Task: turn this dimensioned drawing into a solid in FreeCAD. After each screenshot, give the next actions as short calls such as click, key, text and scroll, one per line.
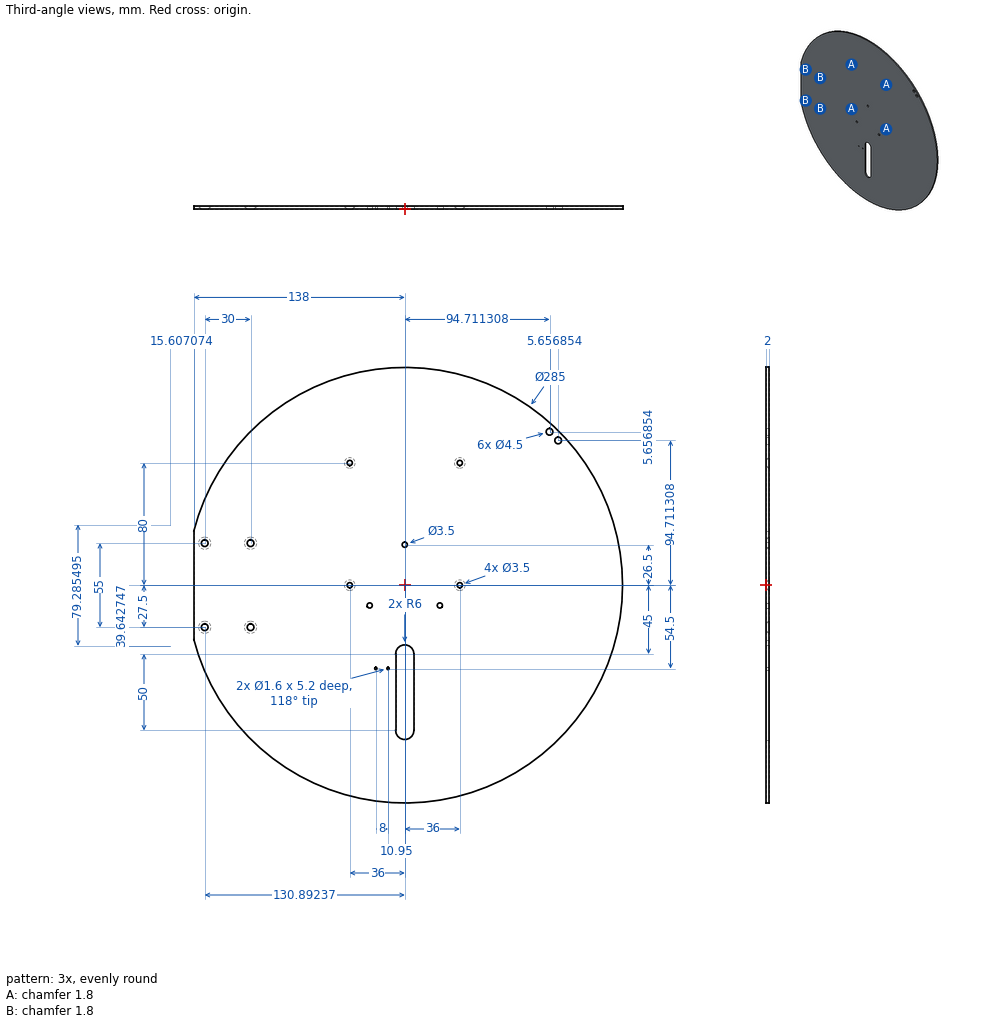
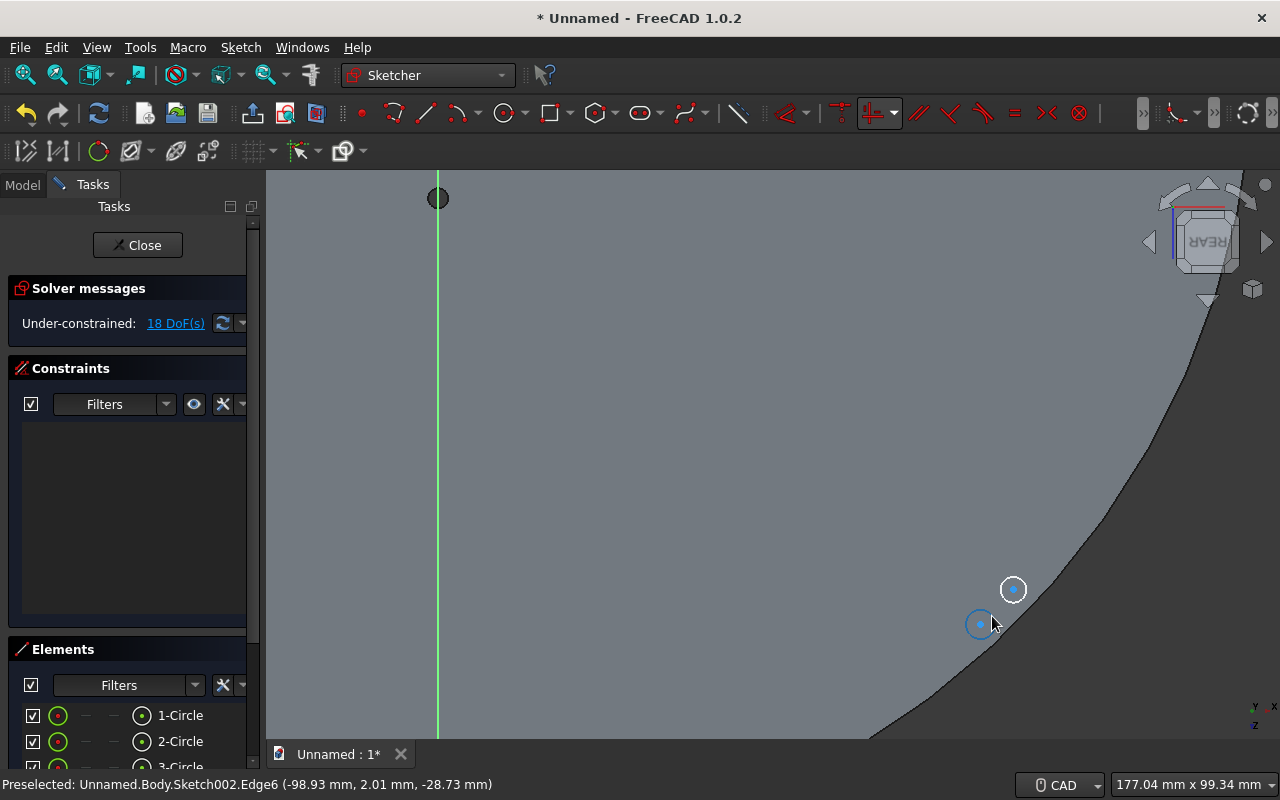
click(991, 614)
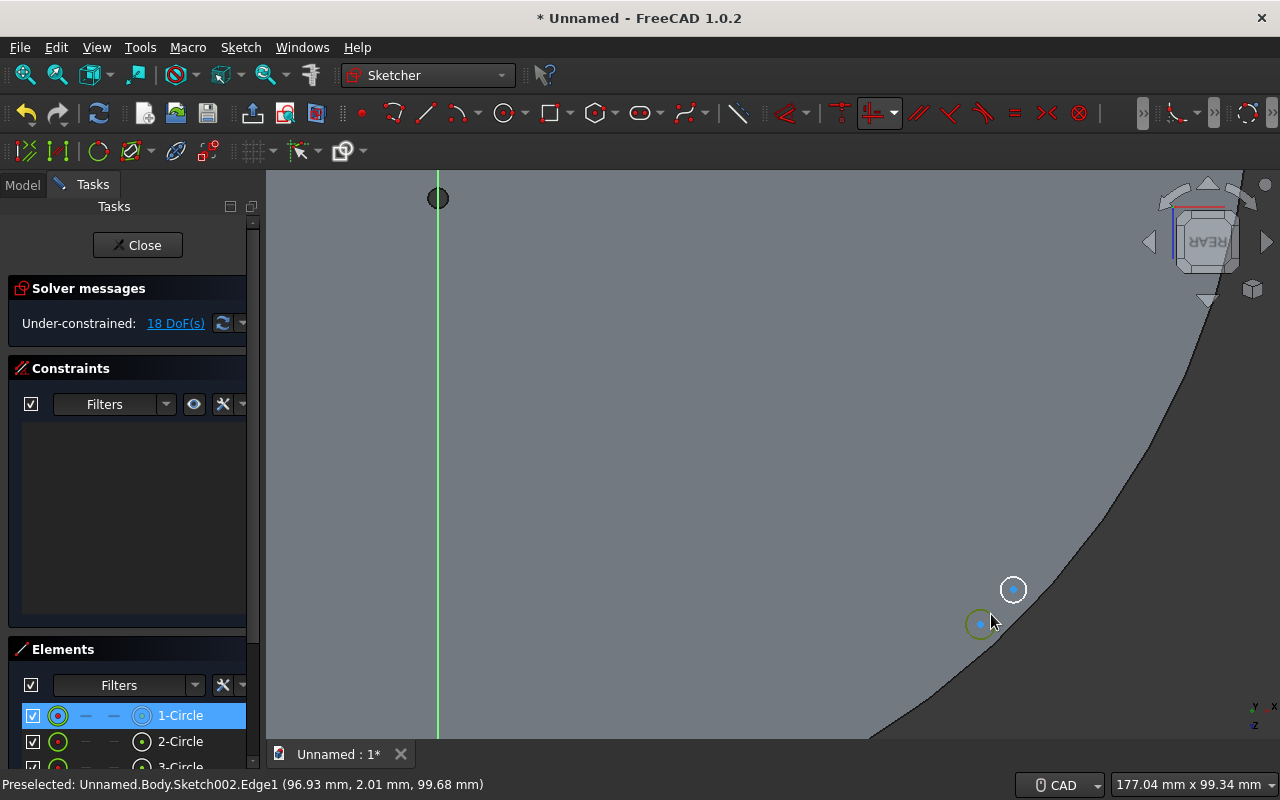
click(1022, 581)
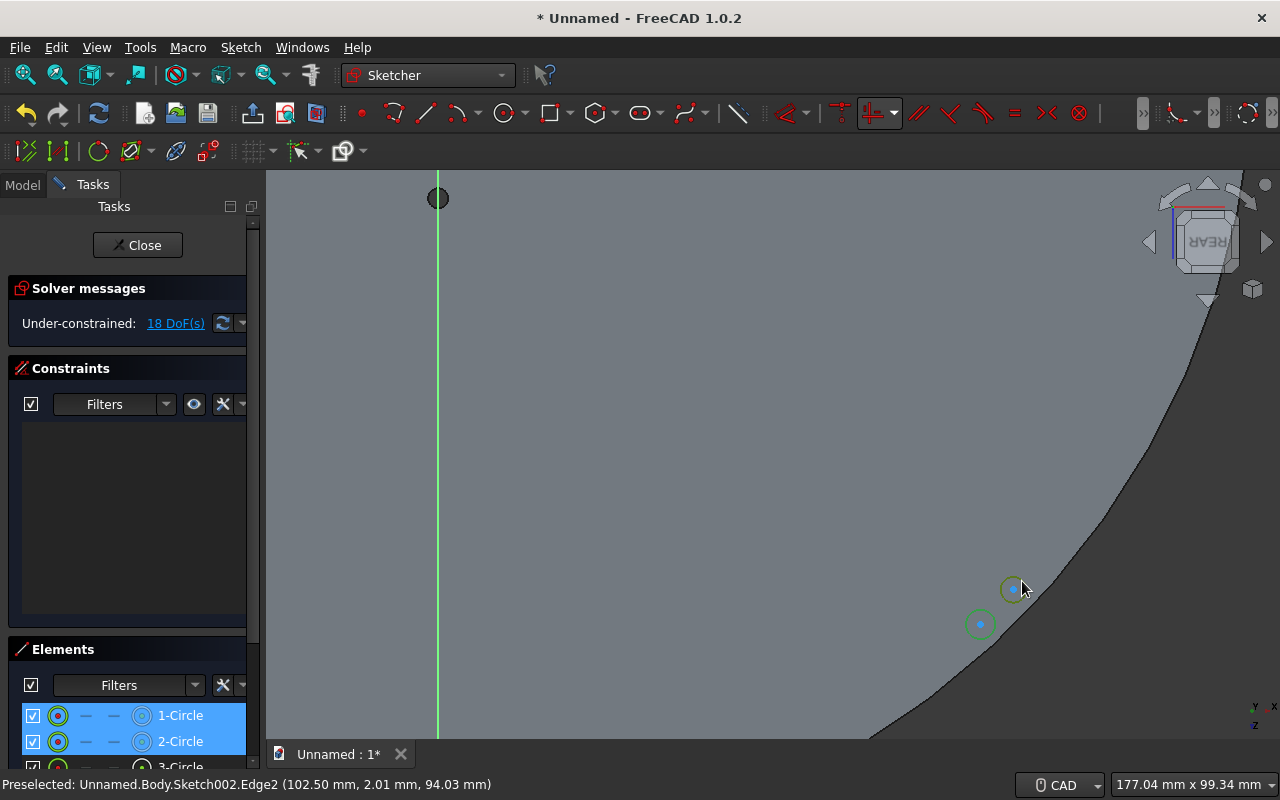
scroll(993, 617, down, 4)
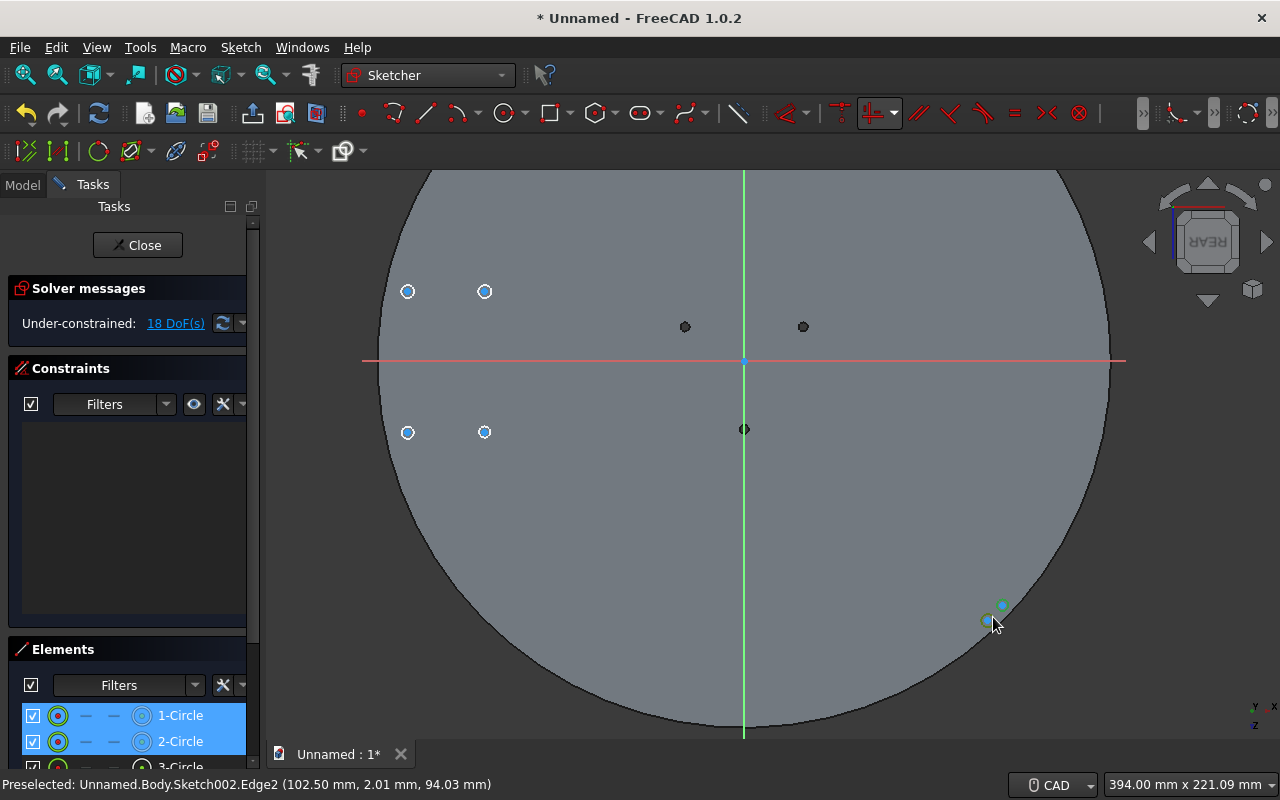
scroll(412, 287, up, 4)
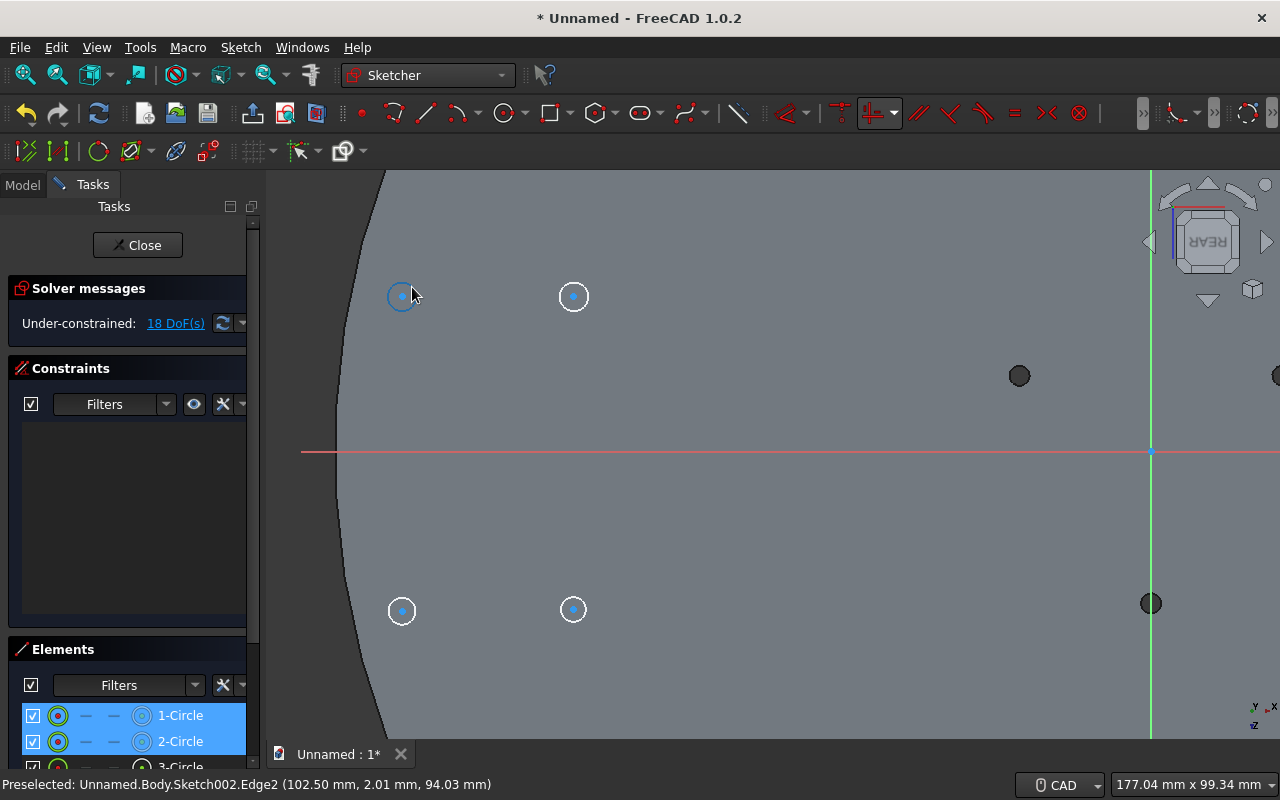
click(412, 287)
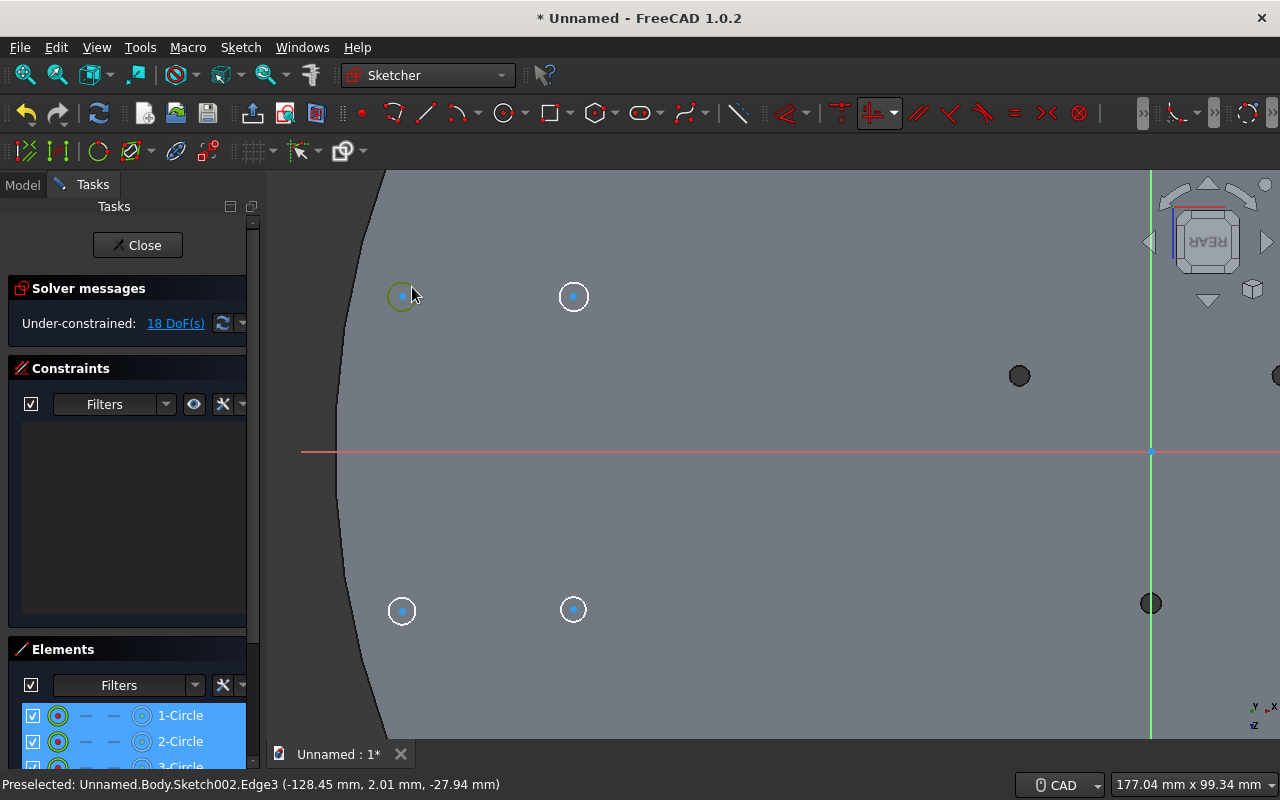
click(412, 602)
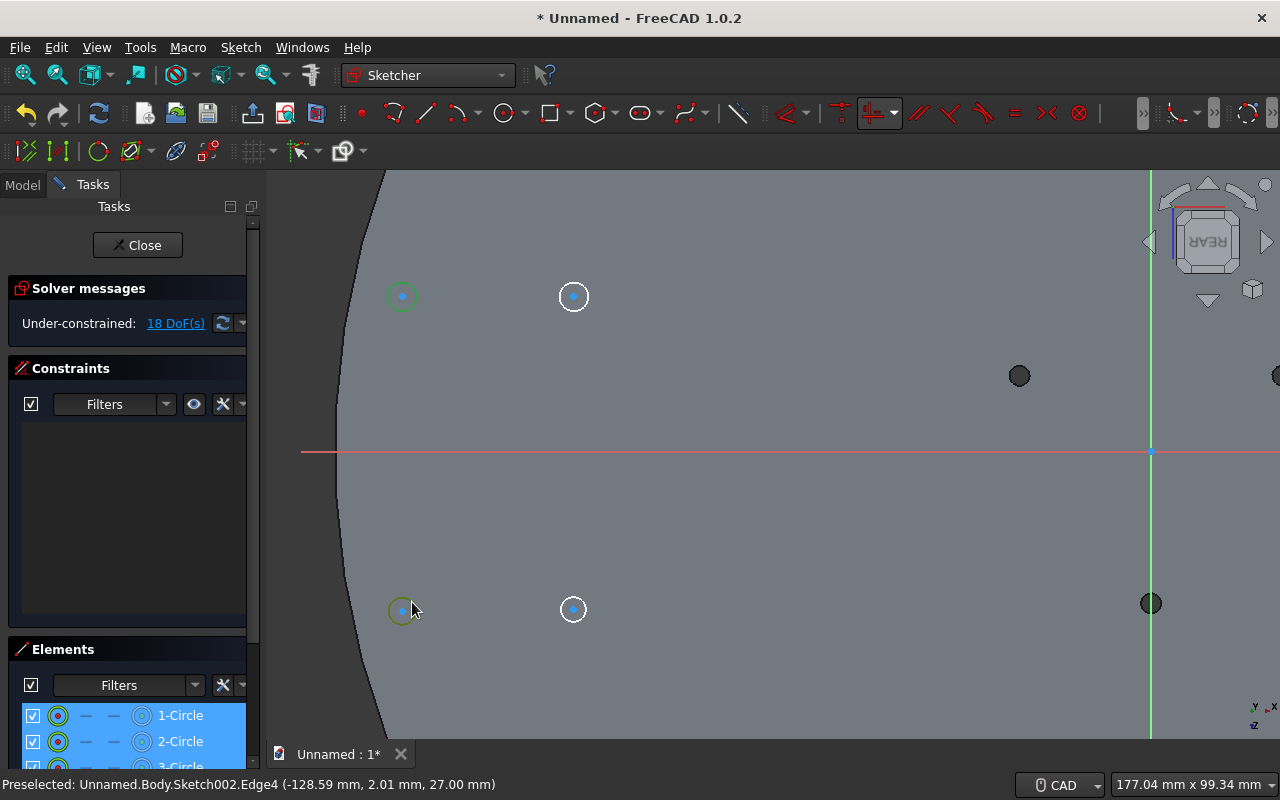
click(582, 601)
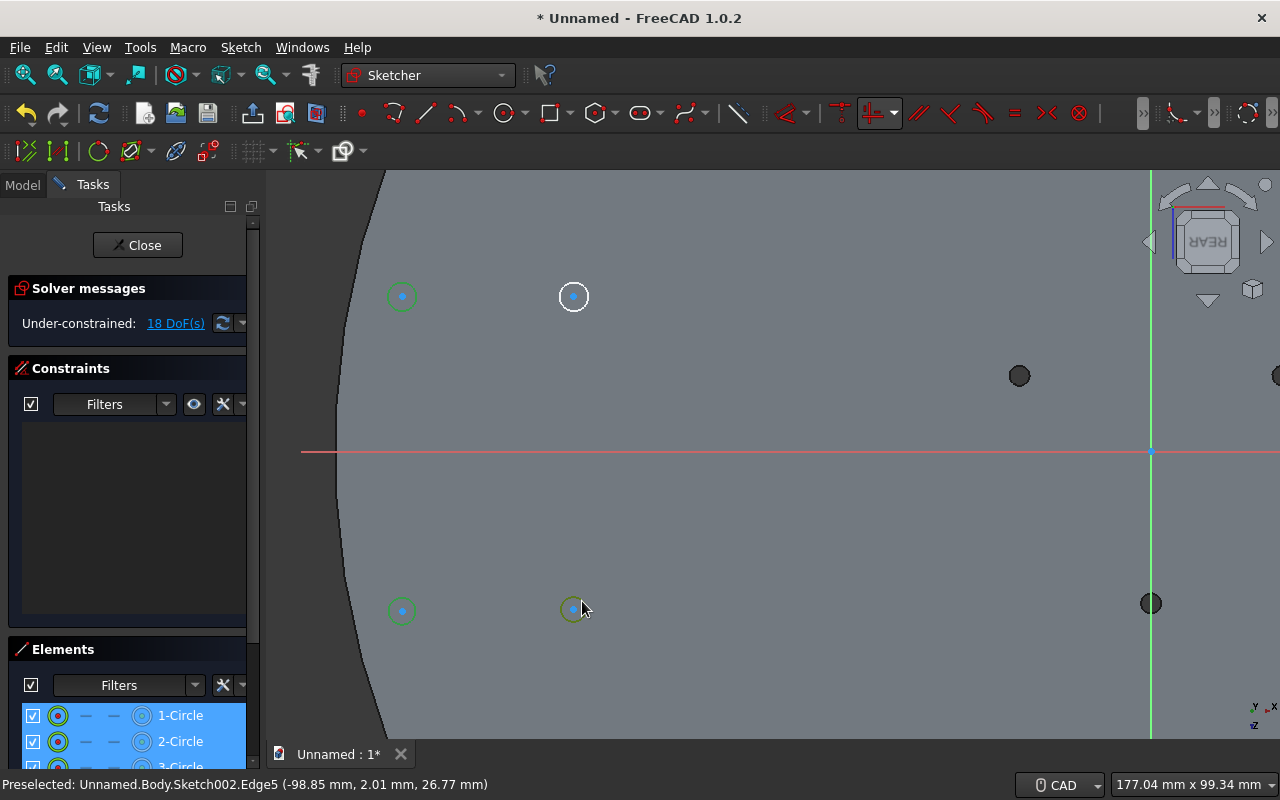
click(584, 287)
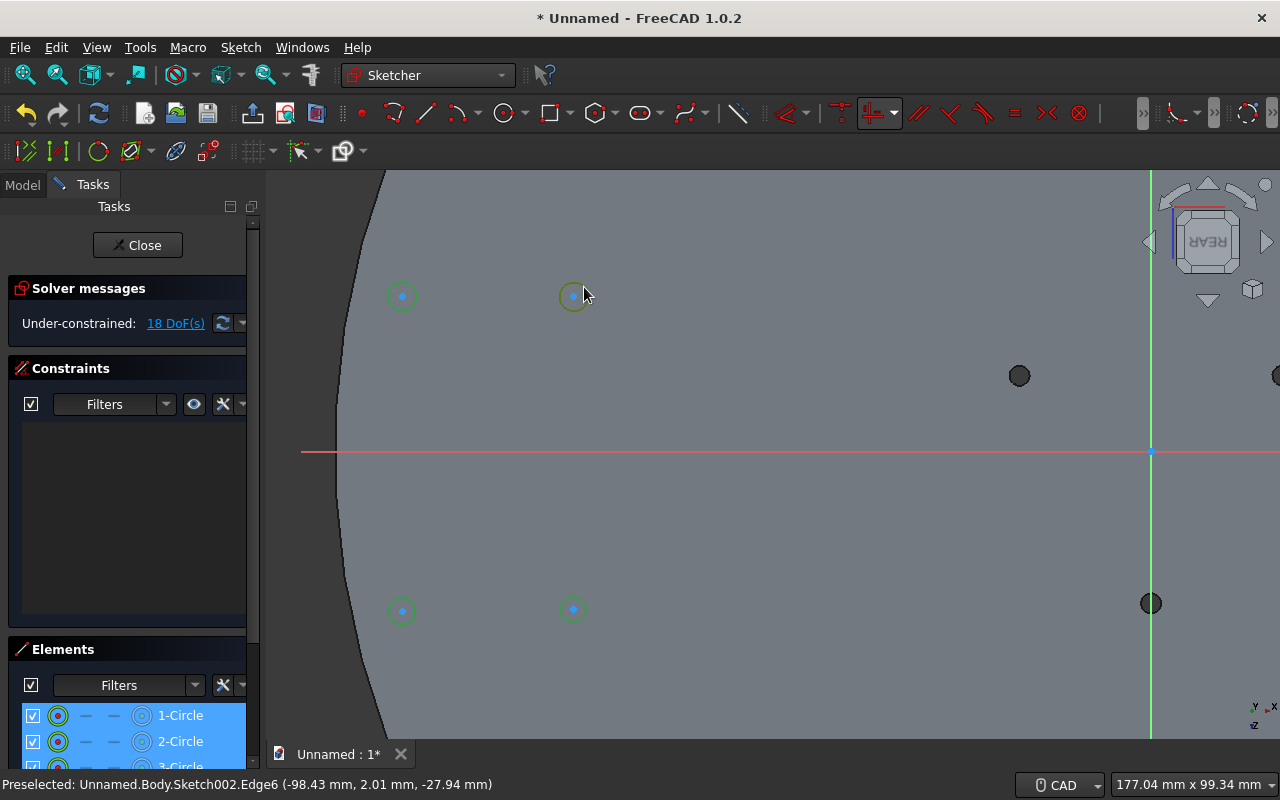
key(e)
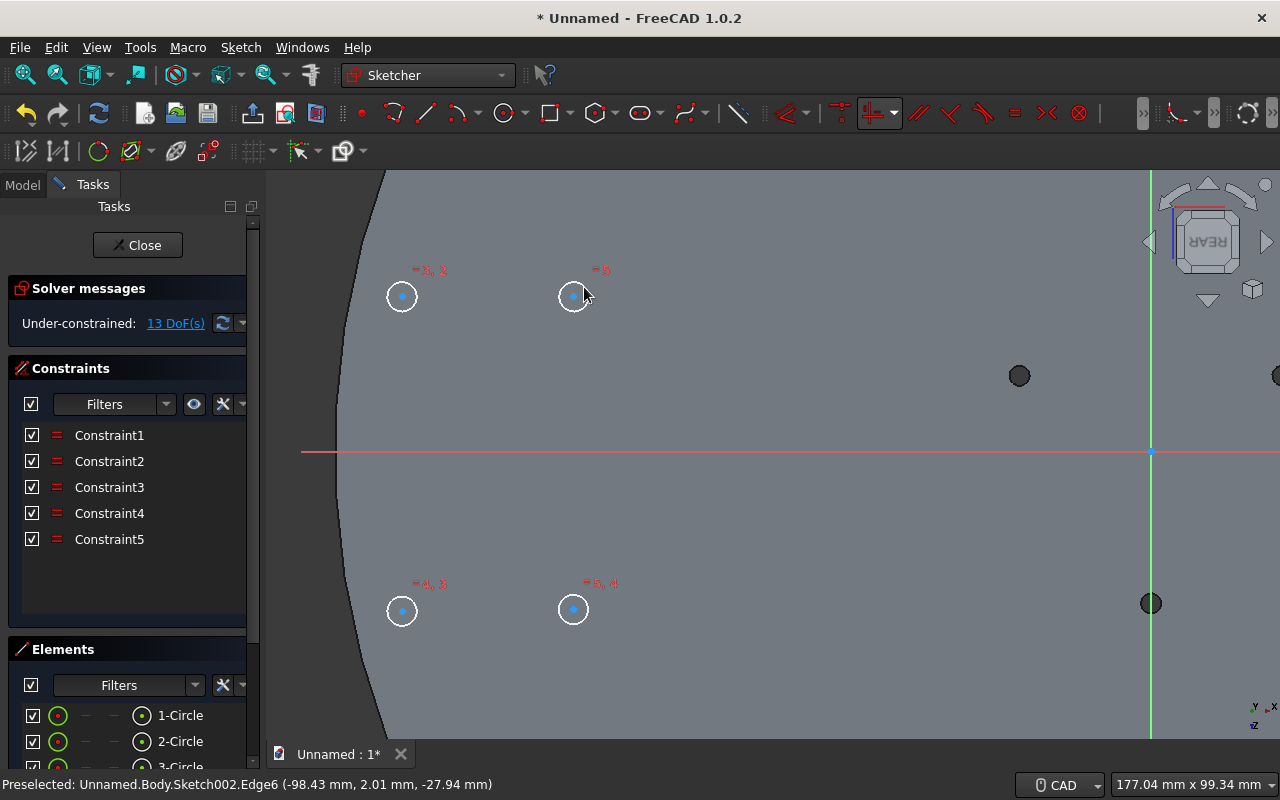
click(402, 297)